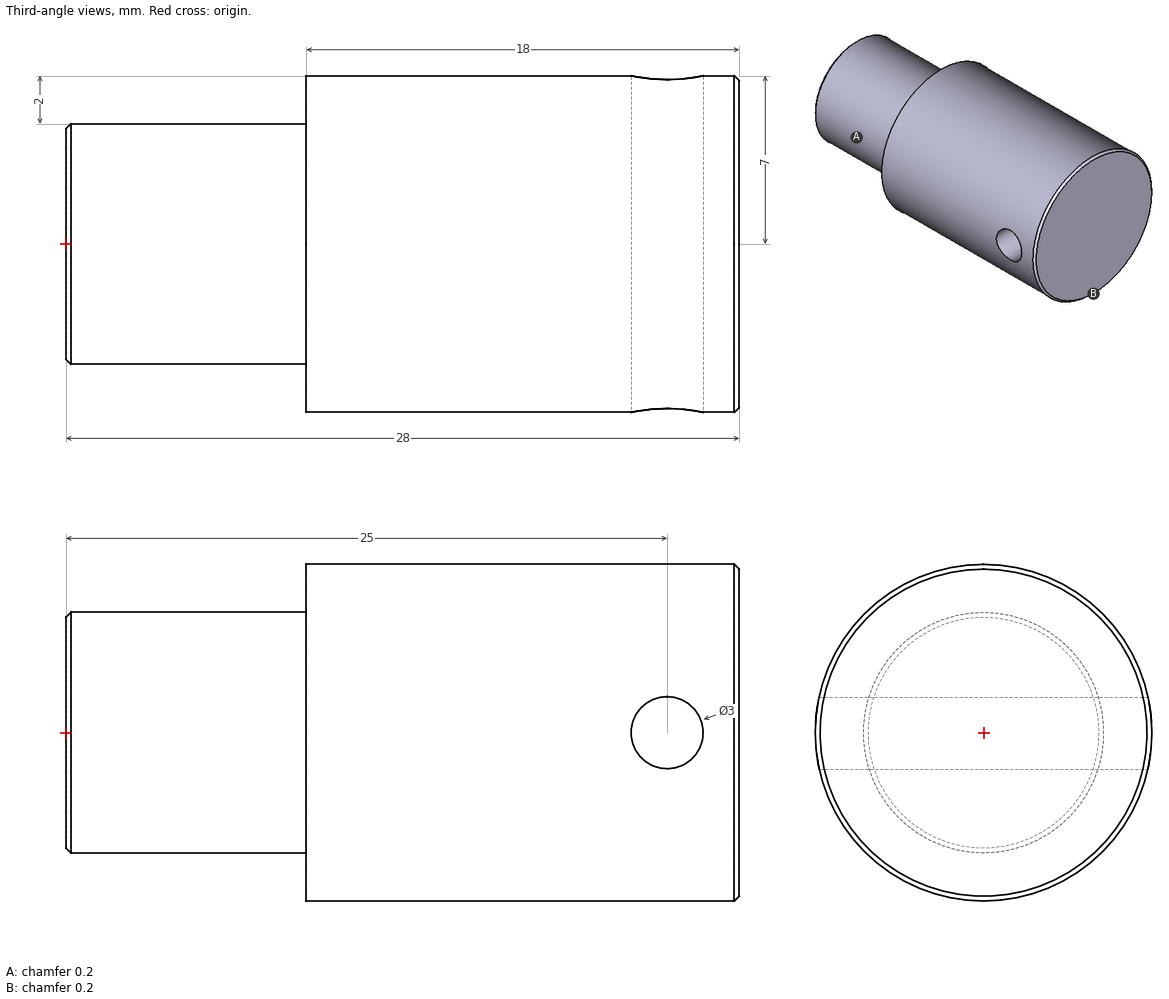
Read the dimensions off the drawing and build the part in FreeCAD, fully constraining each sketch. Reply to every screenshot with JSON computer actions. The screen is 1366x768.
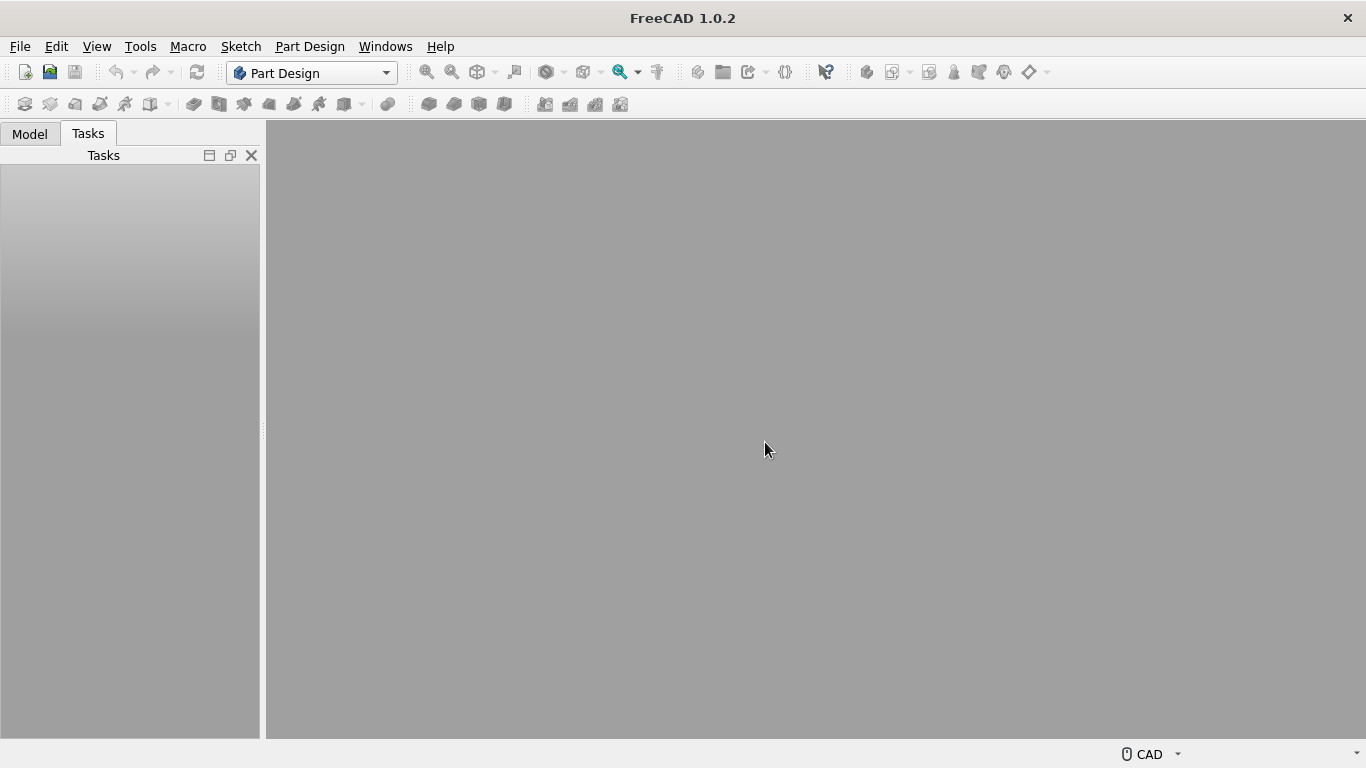
{"action": "key", "text": "ctrl+n"}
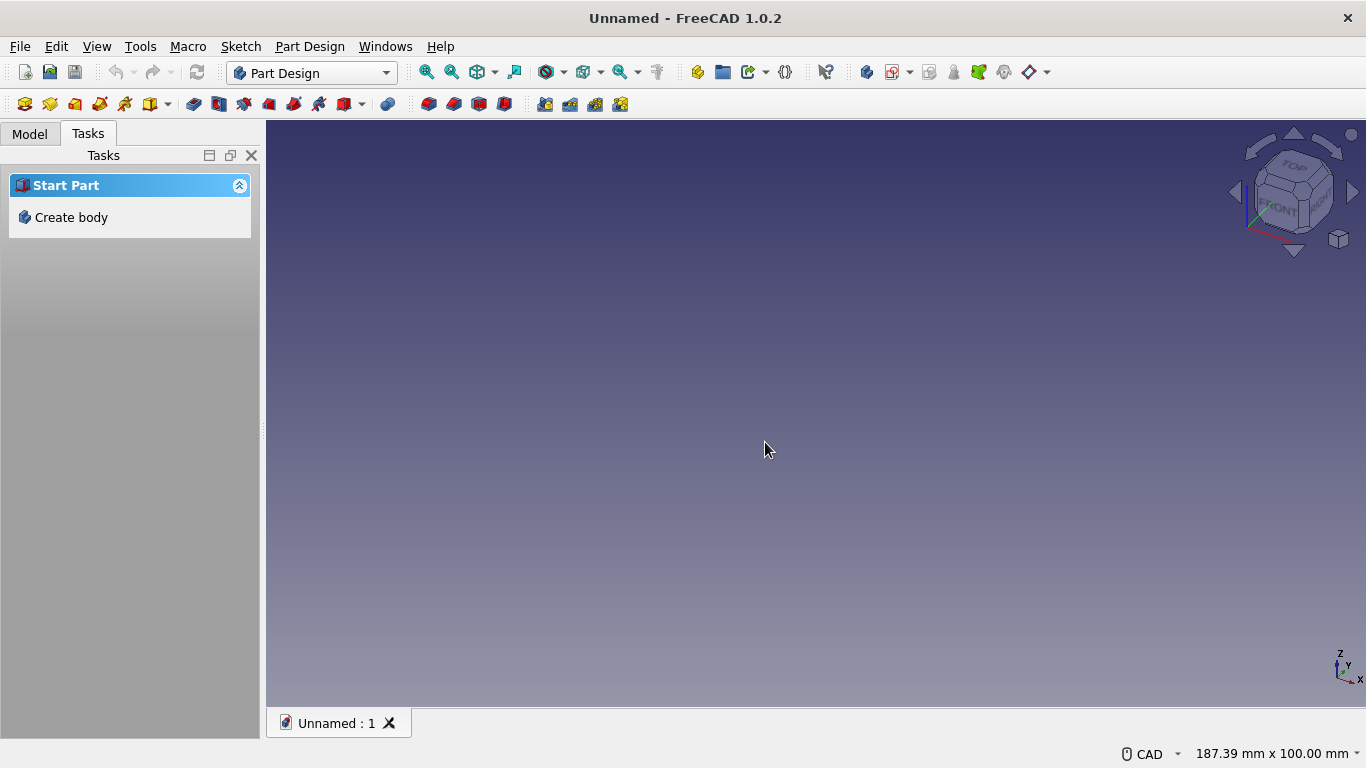
{"action": "left_click", "coordinate": [892, 72]}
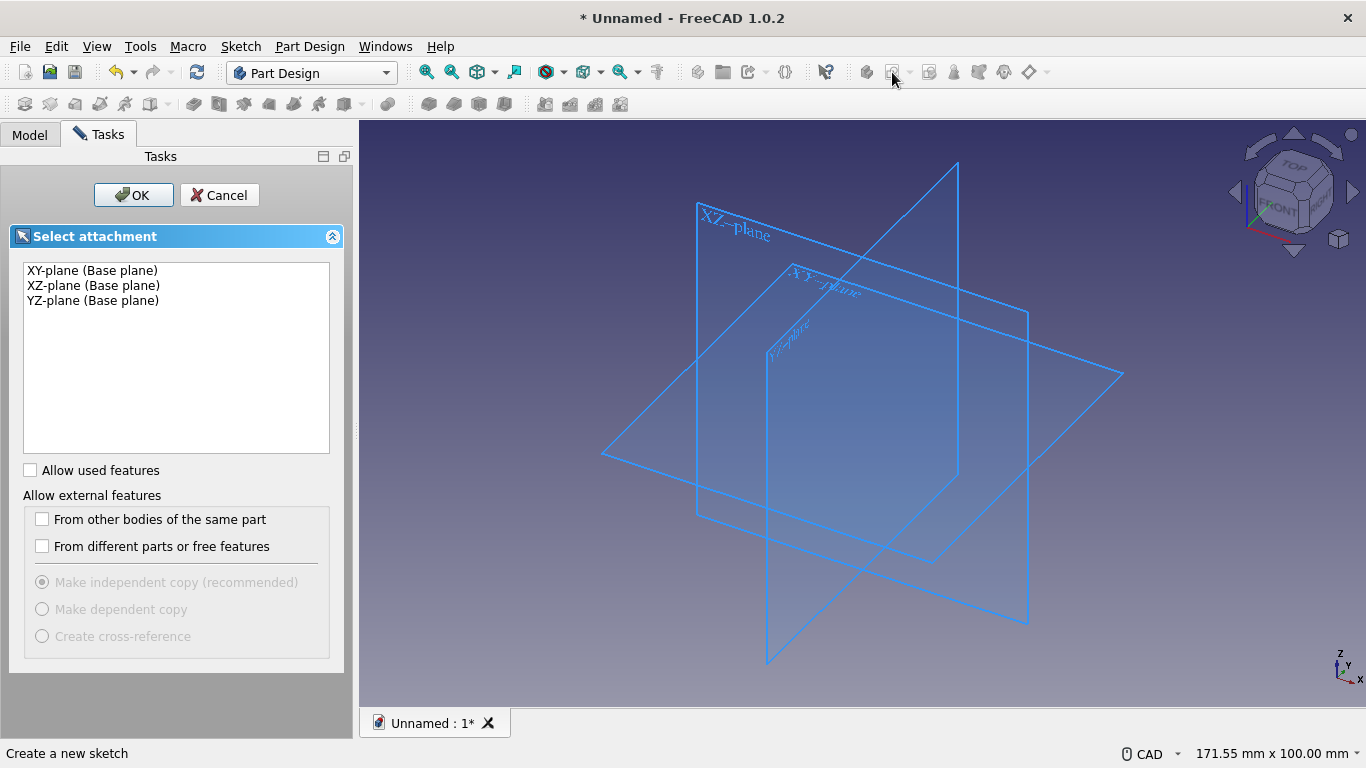
{"action": "left_click", "coordinate": [84, 270]}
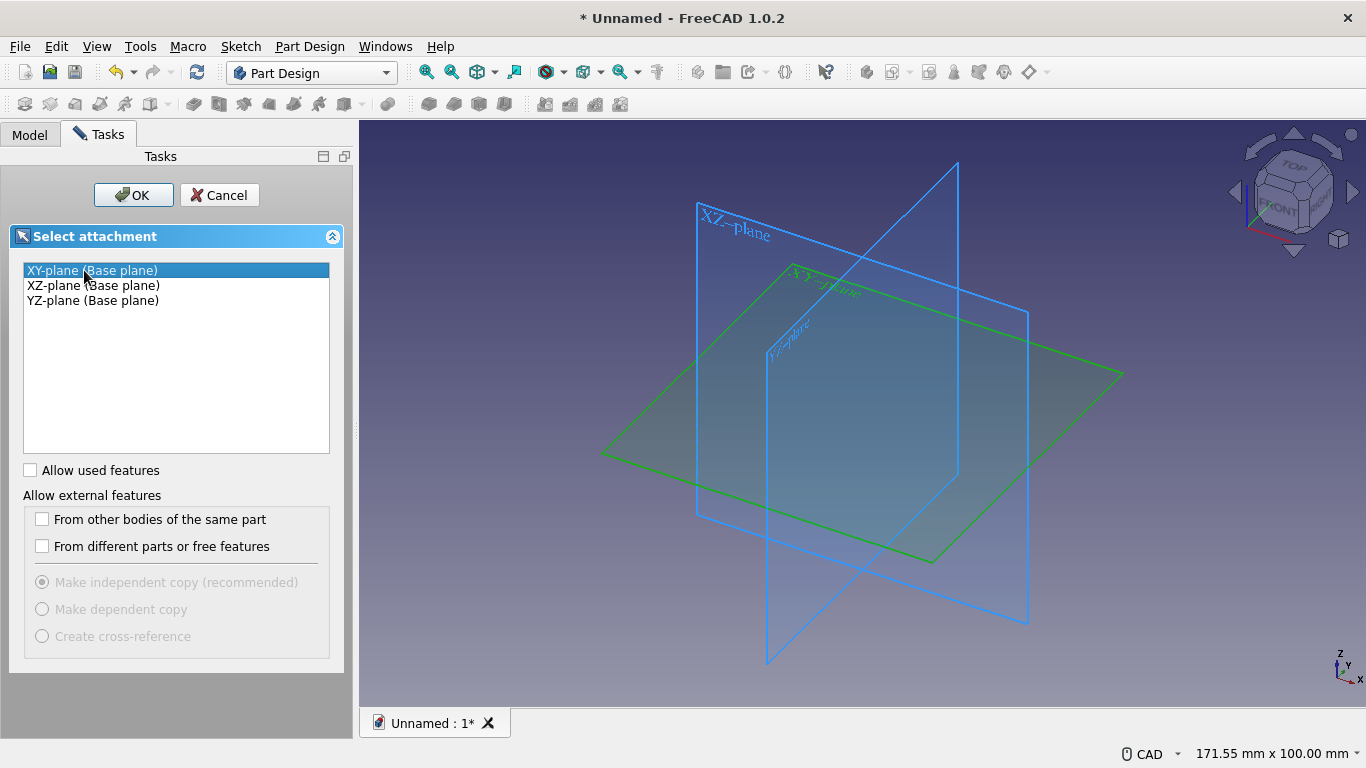
{"action": "left_click", "coordinate": [134, 195]}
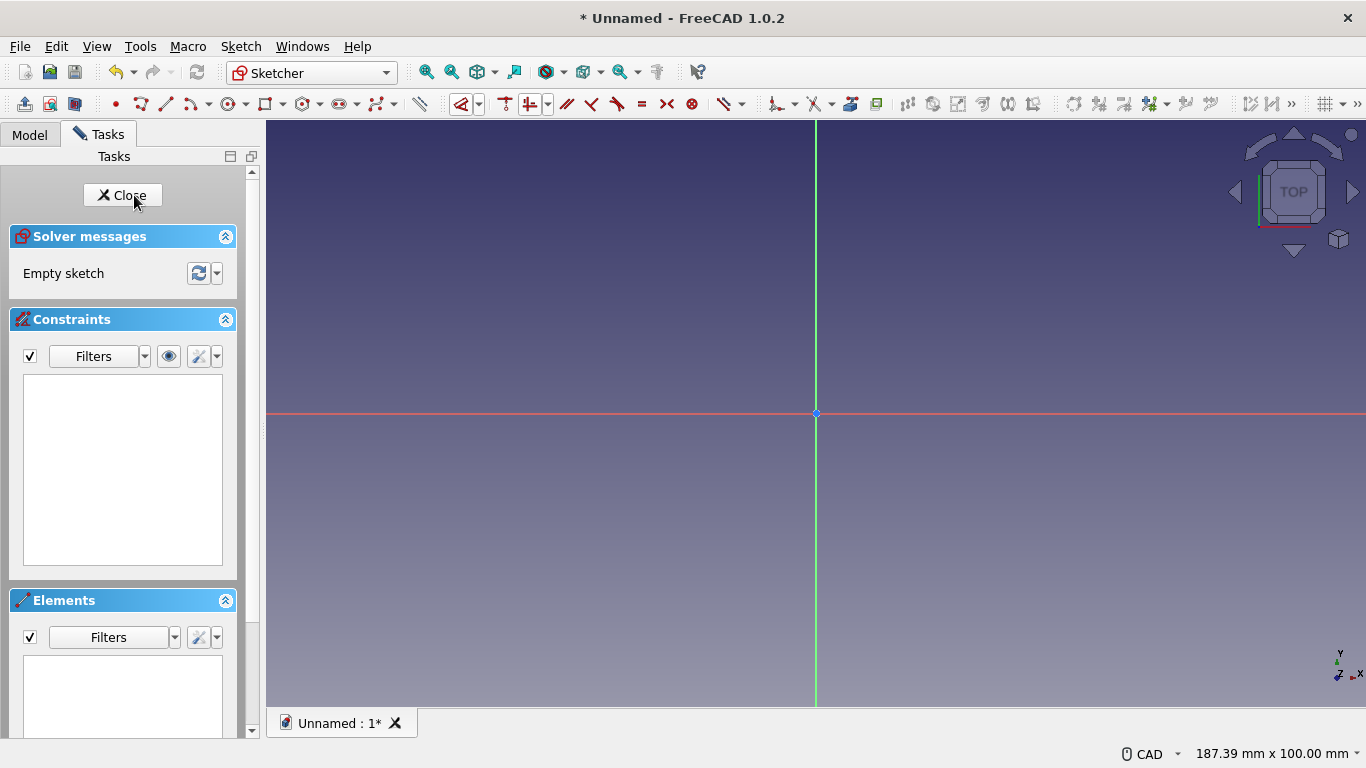
{"action": "scroll", "coordinate": [947, 386], "scroll_direction": "up", "scroll_amount": 7}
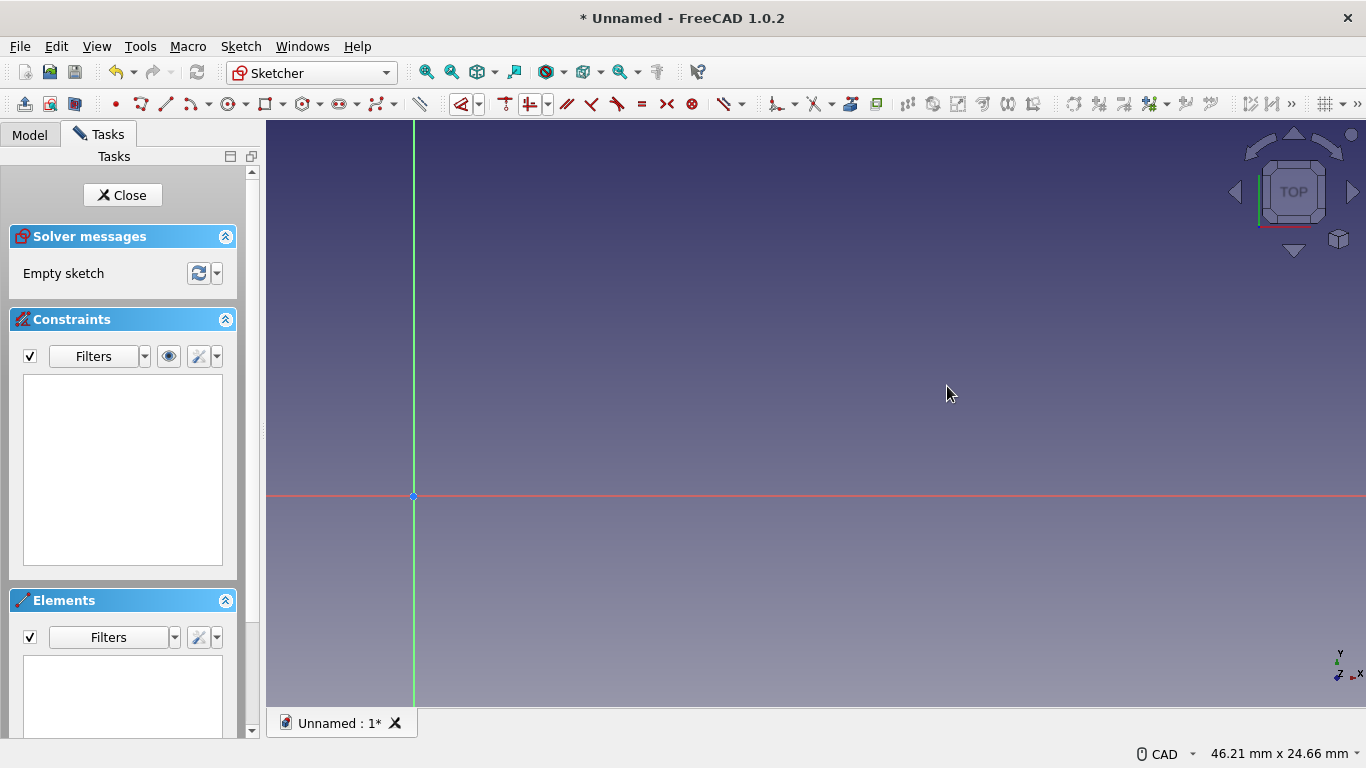
{"action": "key", "text": "g m"}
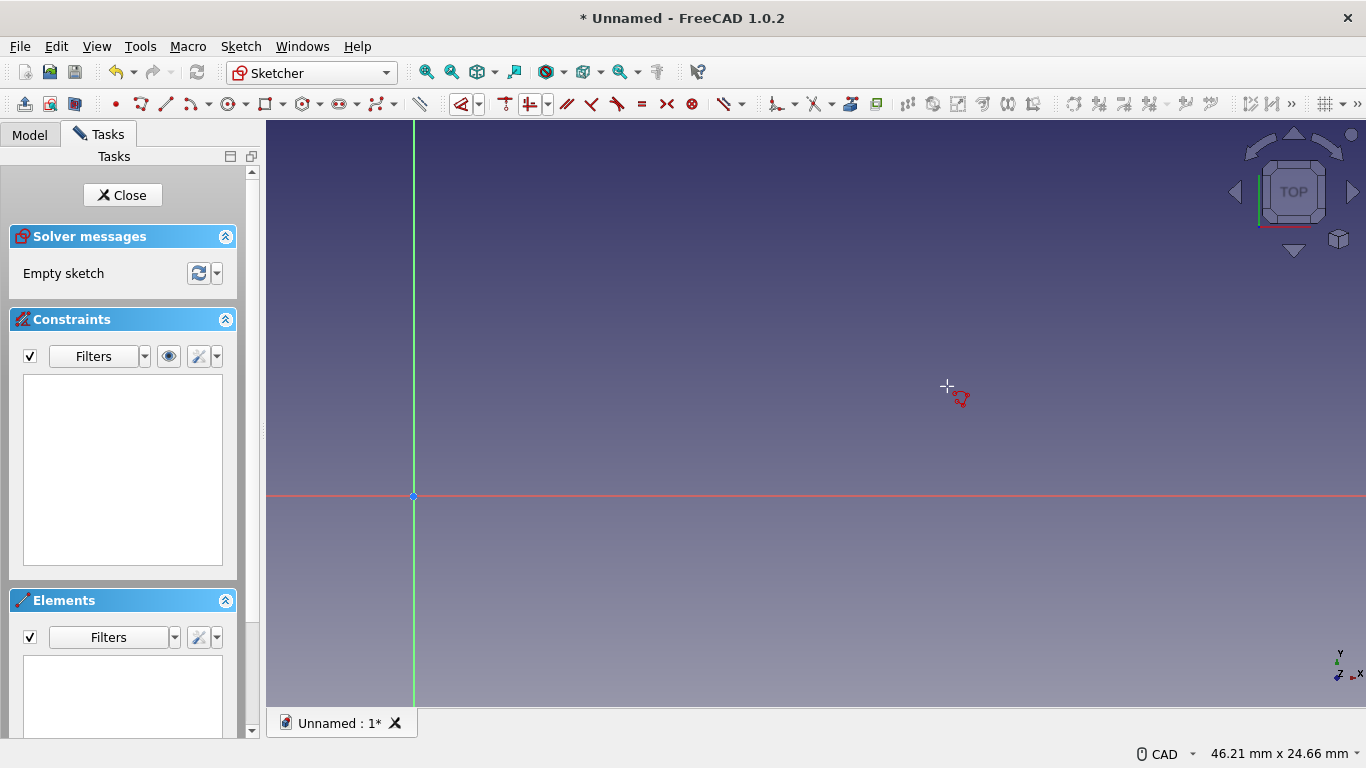
{"action": "left_click", "coordinate": [414, 496]}
{"action": "left_click", "coordinate": [1080, 487]}
{"action": "left_click", "coordinate": [1080, 330]}
{"action": "left_click", "coordinate": [652, 330]}
{"action": "left_click", "coordinate": [652, 377]}
{"action": "left_click", "coordinate": [423, 377]}
{"action": "left_click", "coordinate": [414, 496]}
{"action": "key", "text": "Escape"}
{"action": "key", "text": "Escape"}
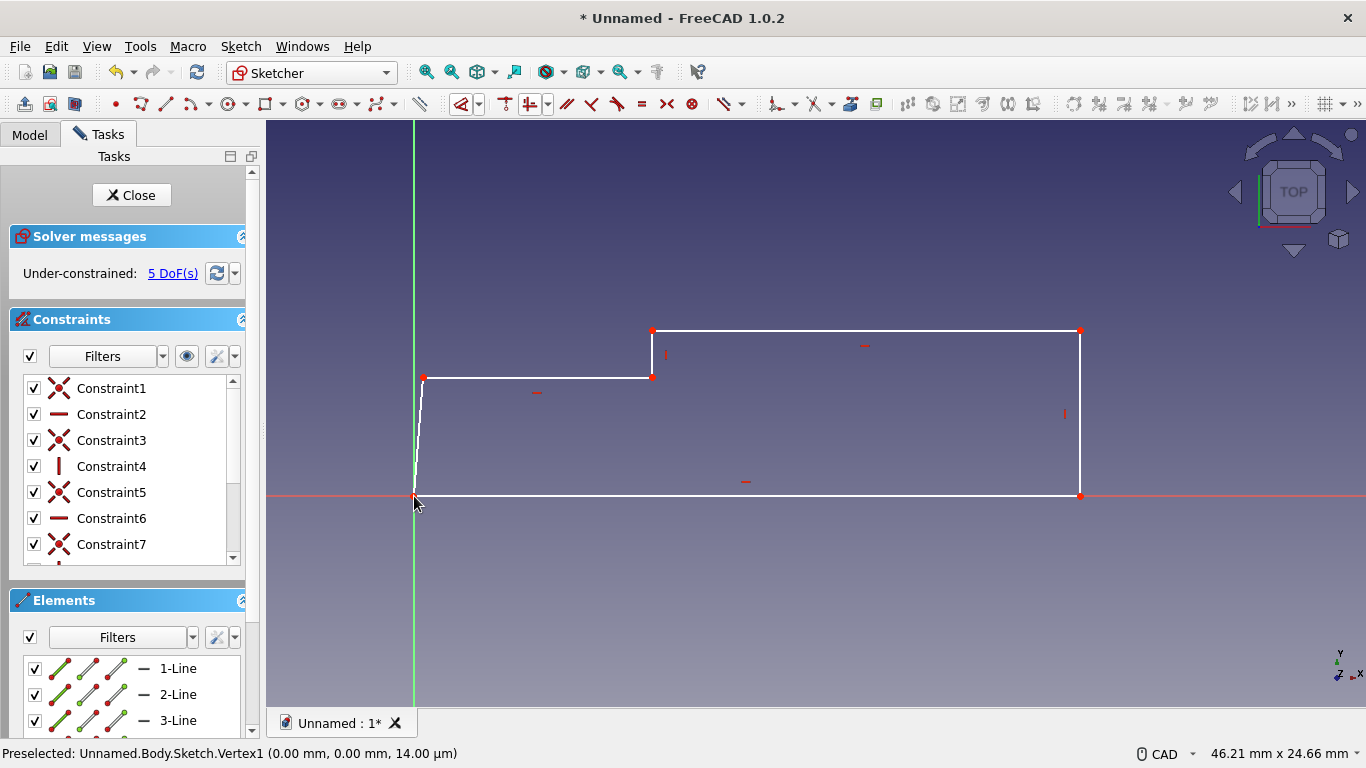
{"action": "left_click", "coordinate": [417, 461]}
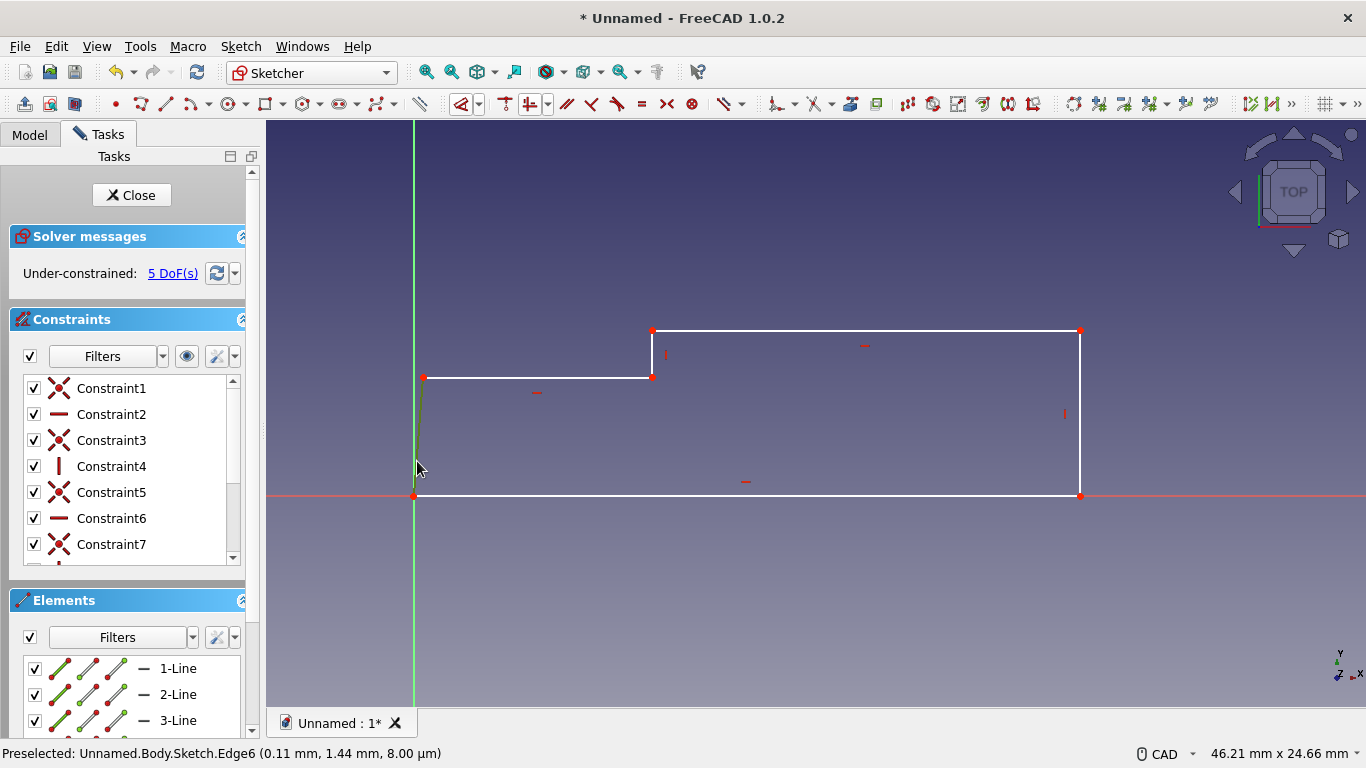
{"action": "key", "text": "v"}